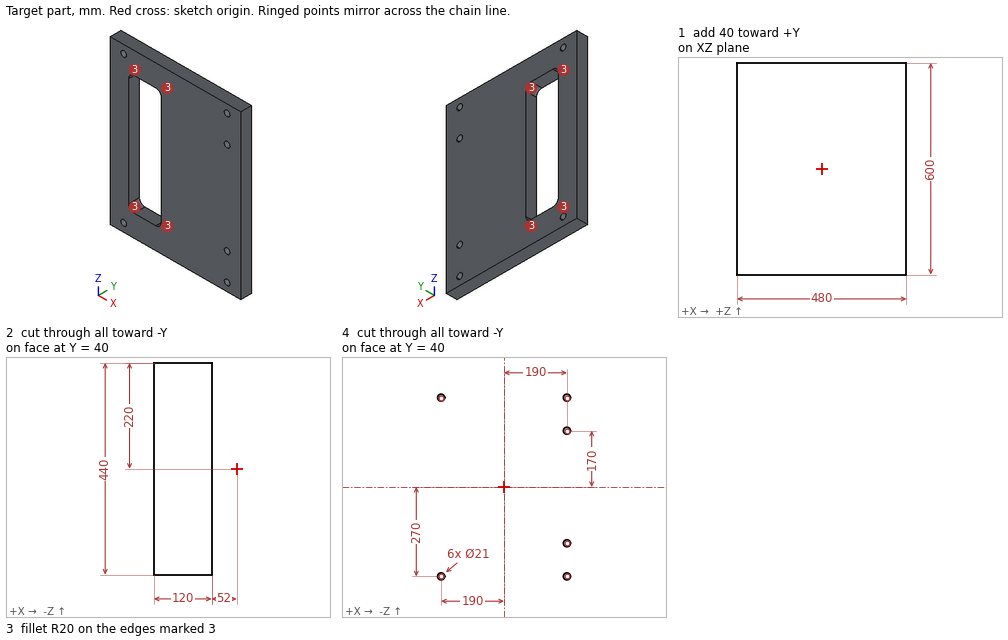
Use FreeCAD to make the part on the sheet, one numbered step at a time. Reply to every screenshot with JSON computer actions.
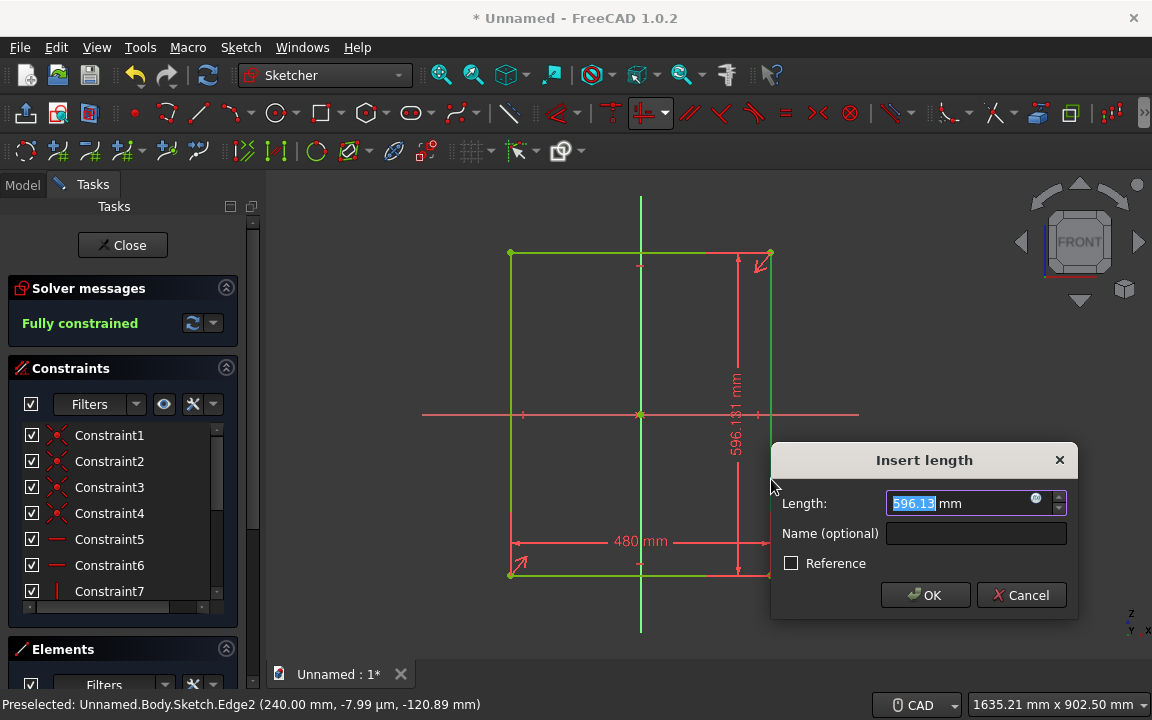
{"action": "type", "text": "600"}
{"action": "key", "text": "Return"}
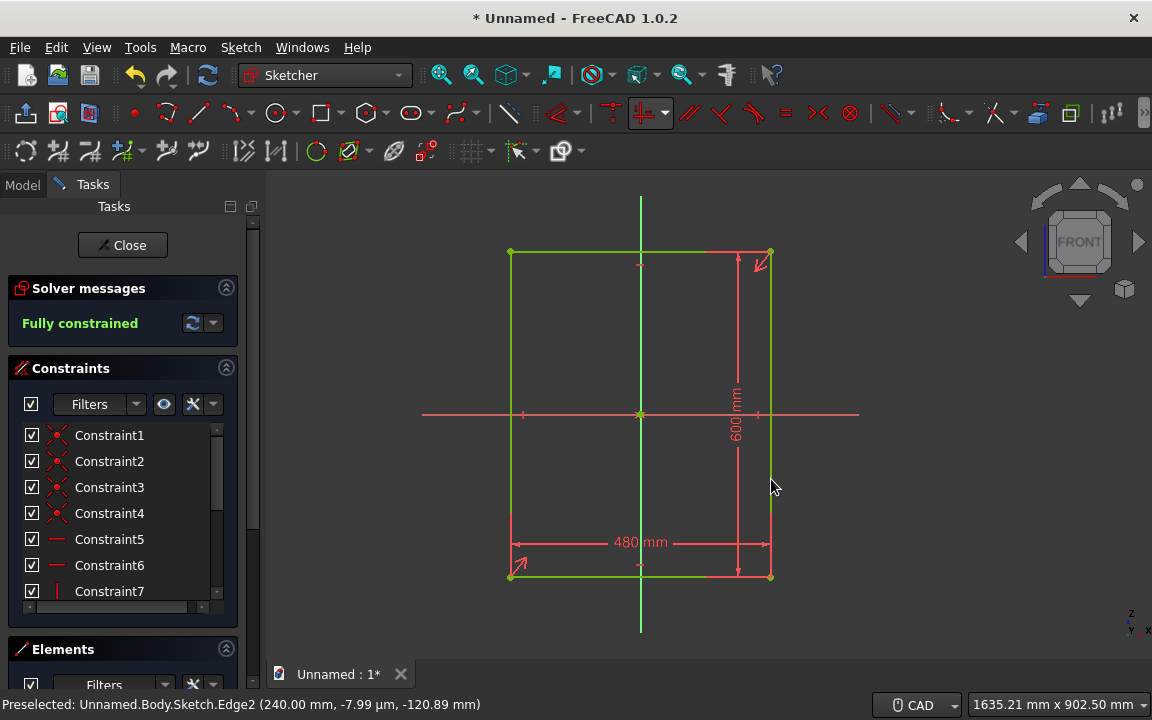
{"action": "left_click", "coordinate": [123, 245]}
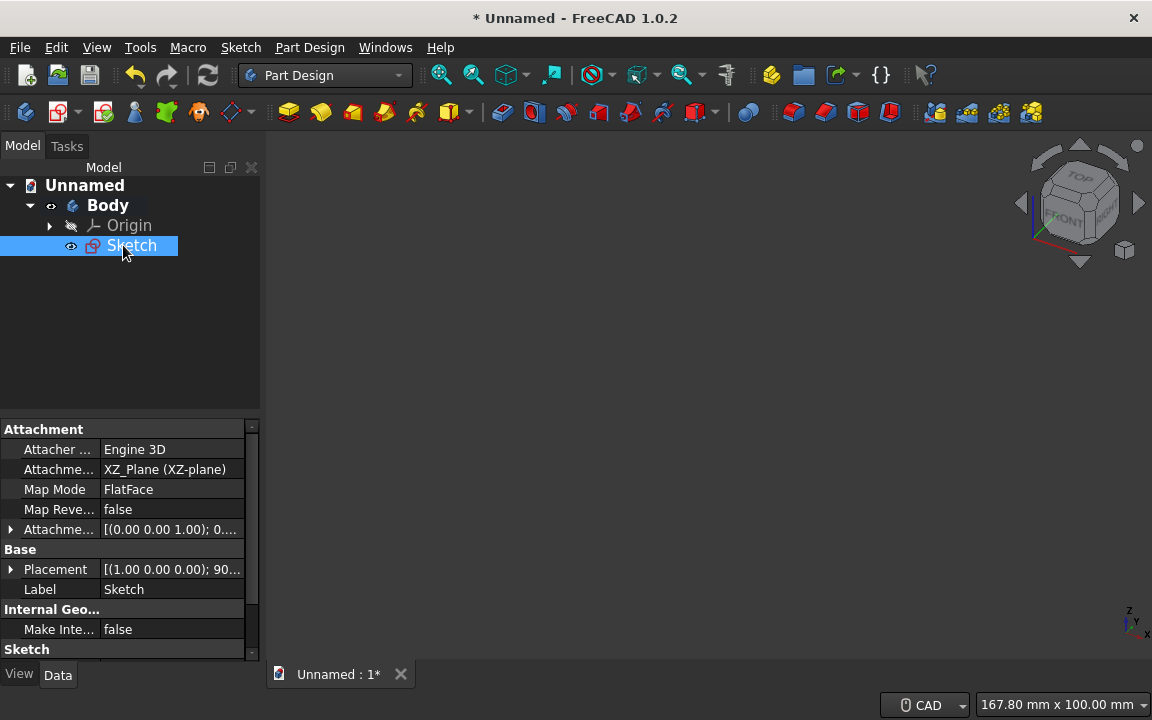
{"action": "left_click", "coordinate": [290, 112]}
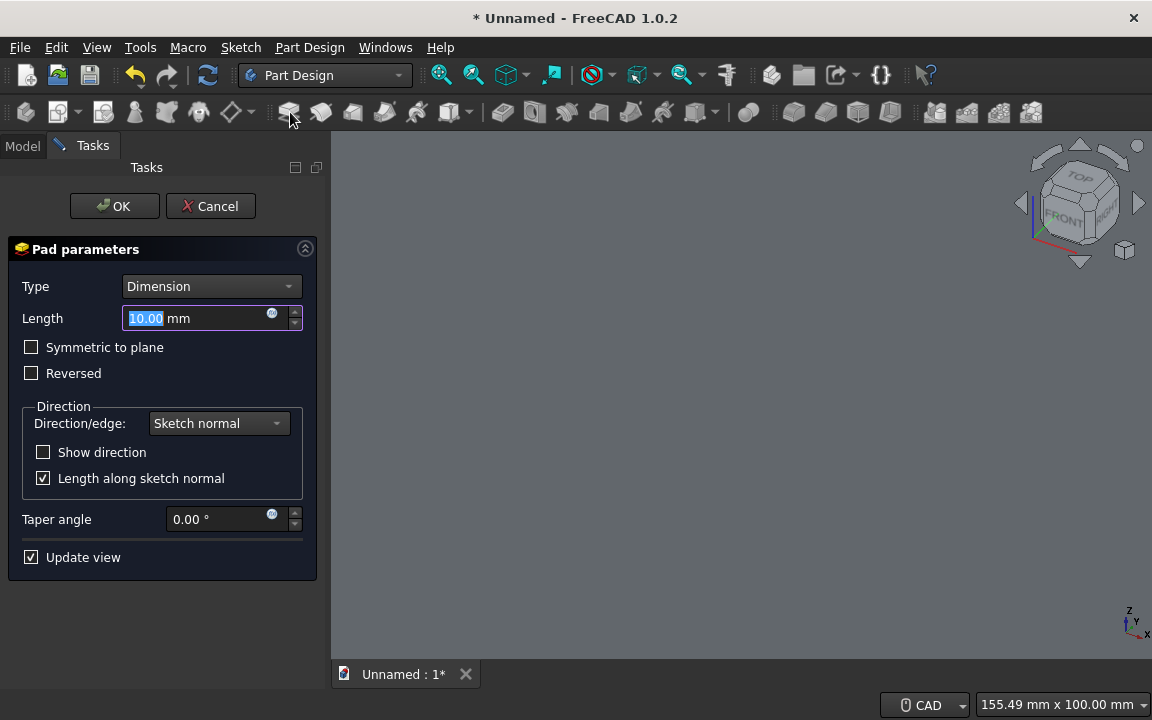
{"action": "type", "text": "40"}
{"action": "key", "text": "Tab"}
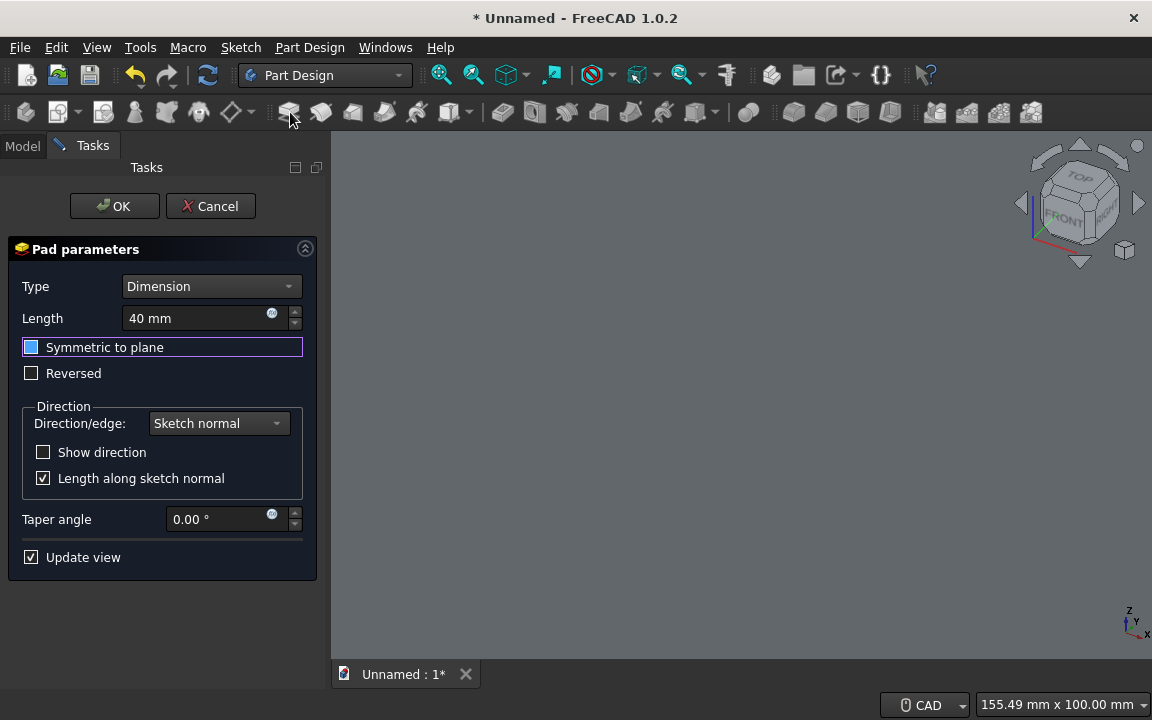
{"action": "left_click", "coordinate": [30, 373]}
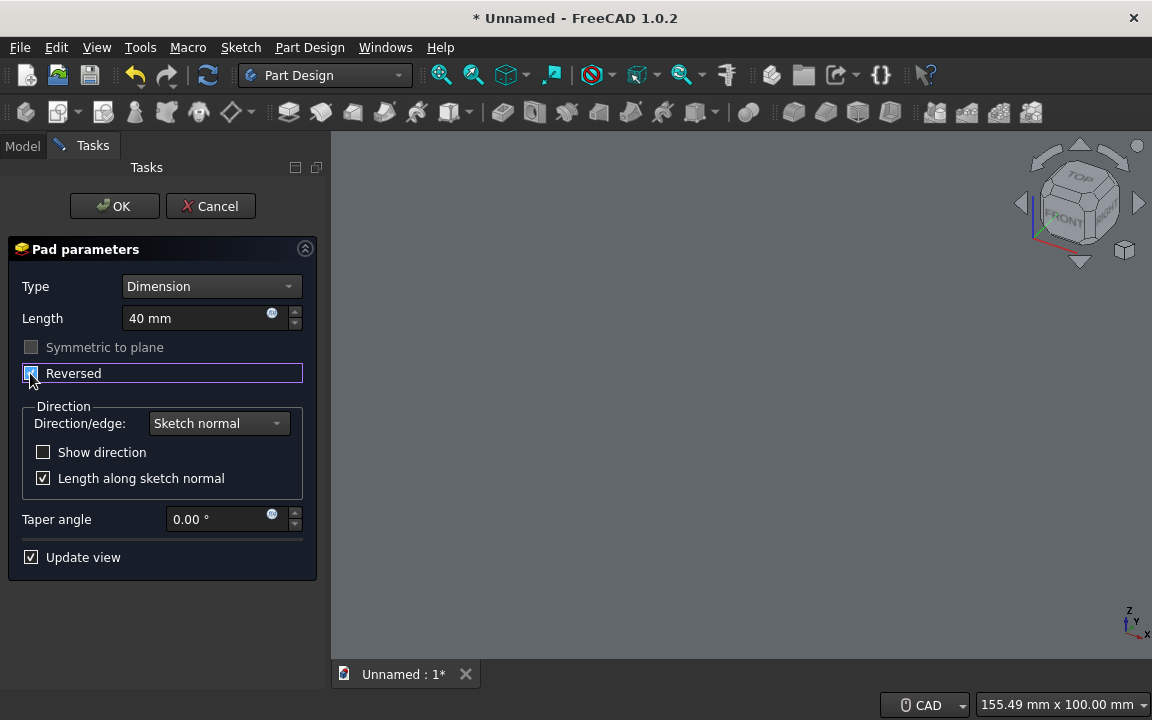
{"action": "left_click", "coordinate": [115, 206]}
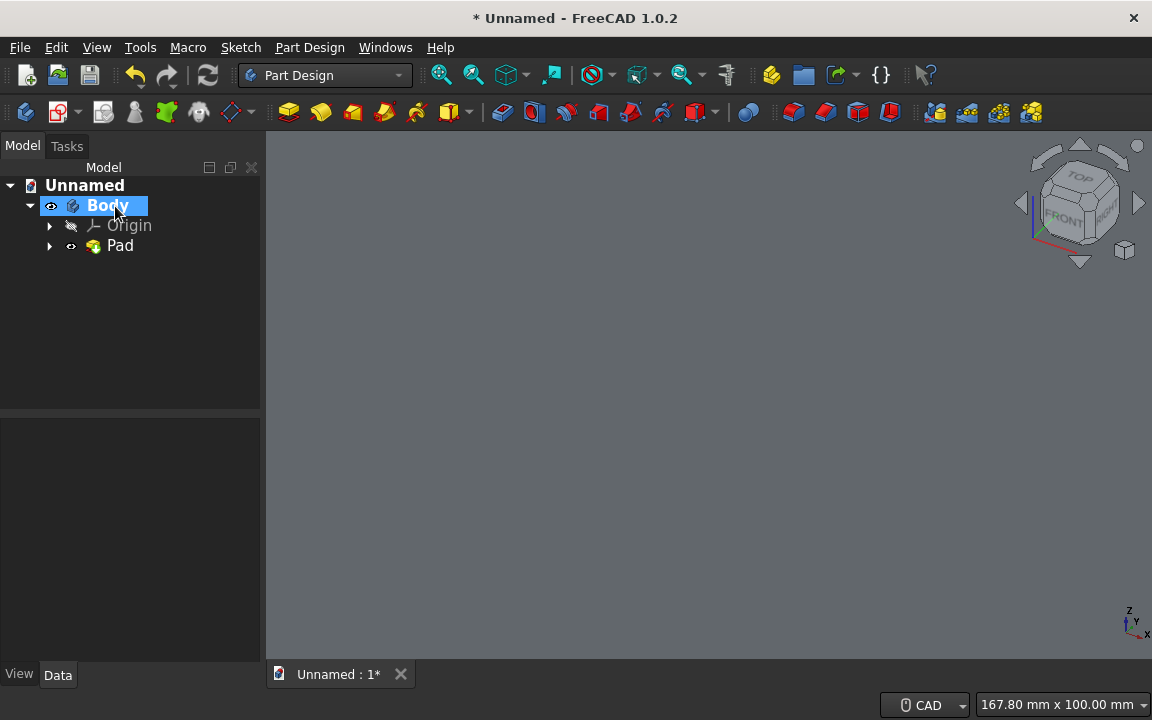
{"action": "key", "text": "v f"}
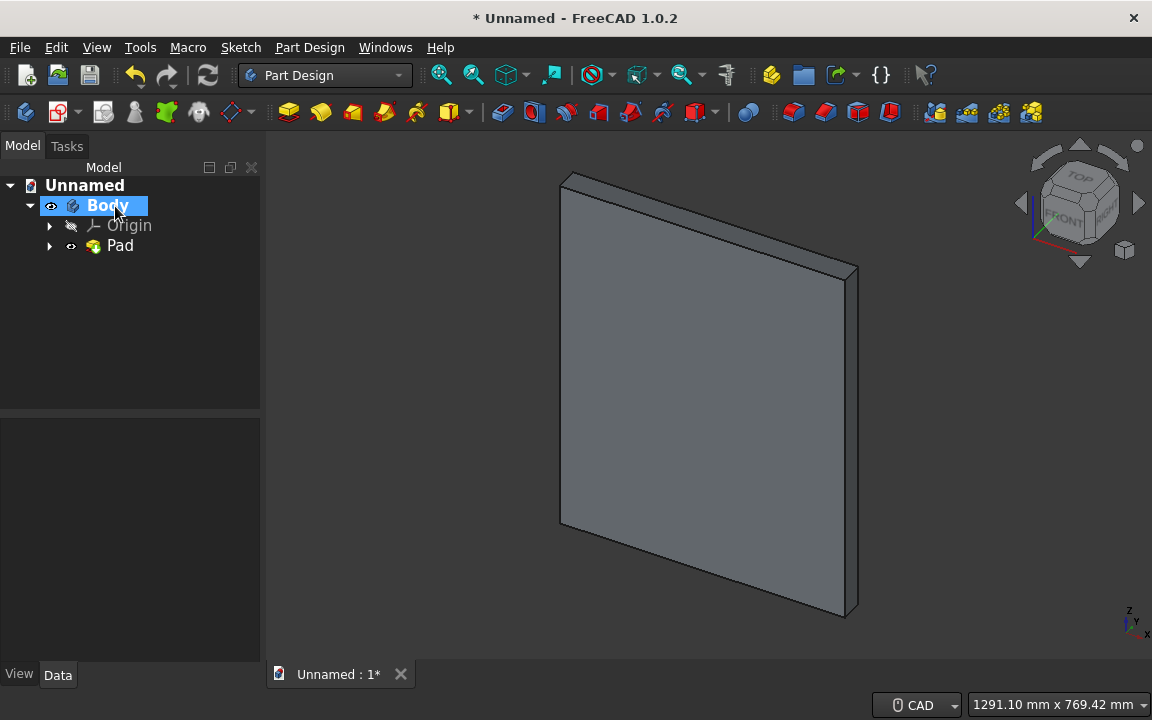
{"action": "key", "text": "4"}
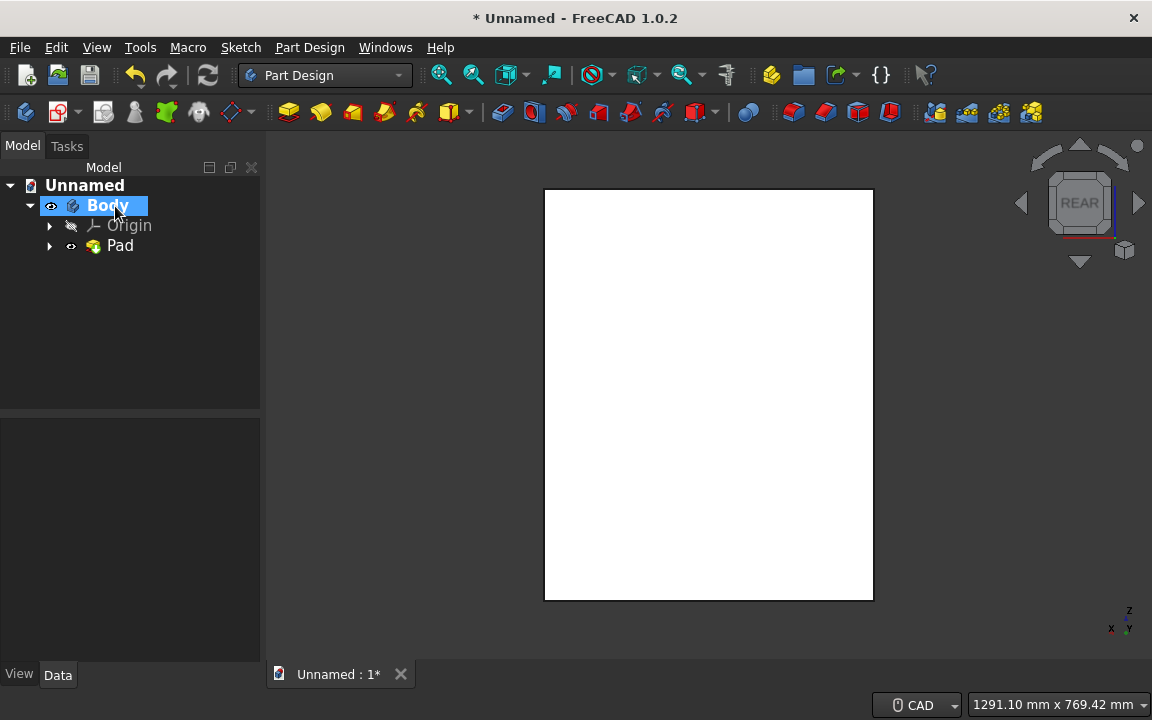
{"action": "left_click", "coordinate": [709, 394]}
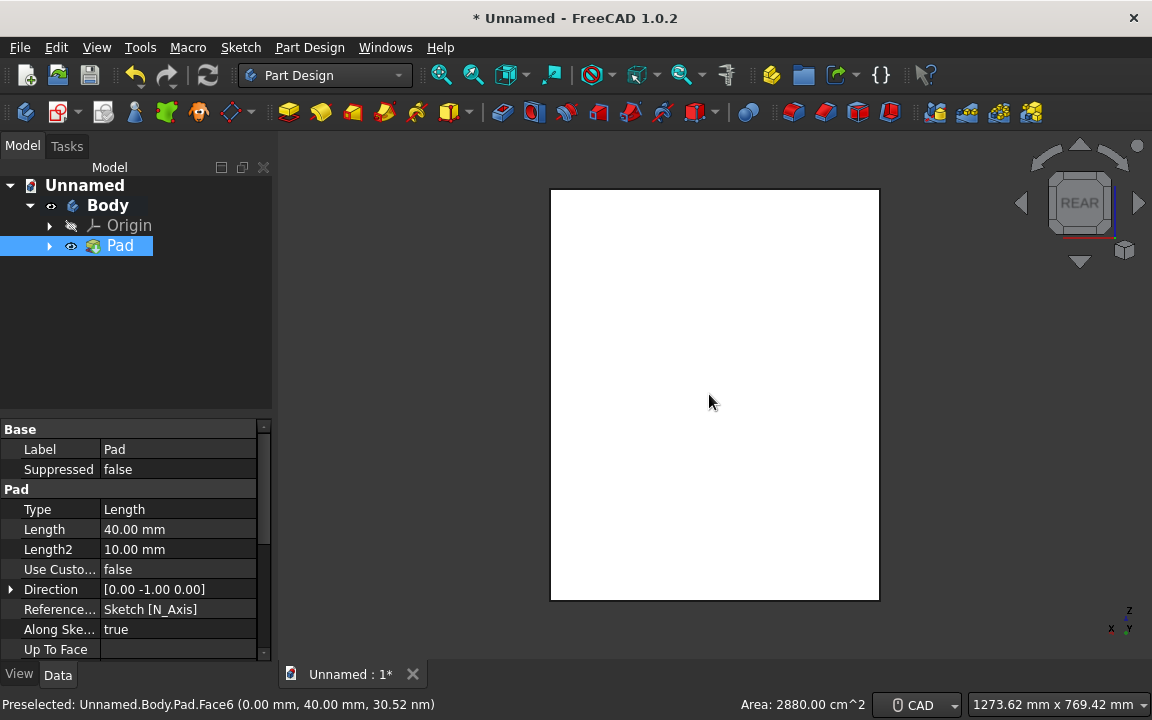
{"action": "left_click", "coordinate": [58, 112]}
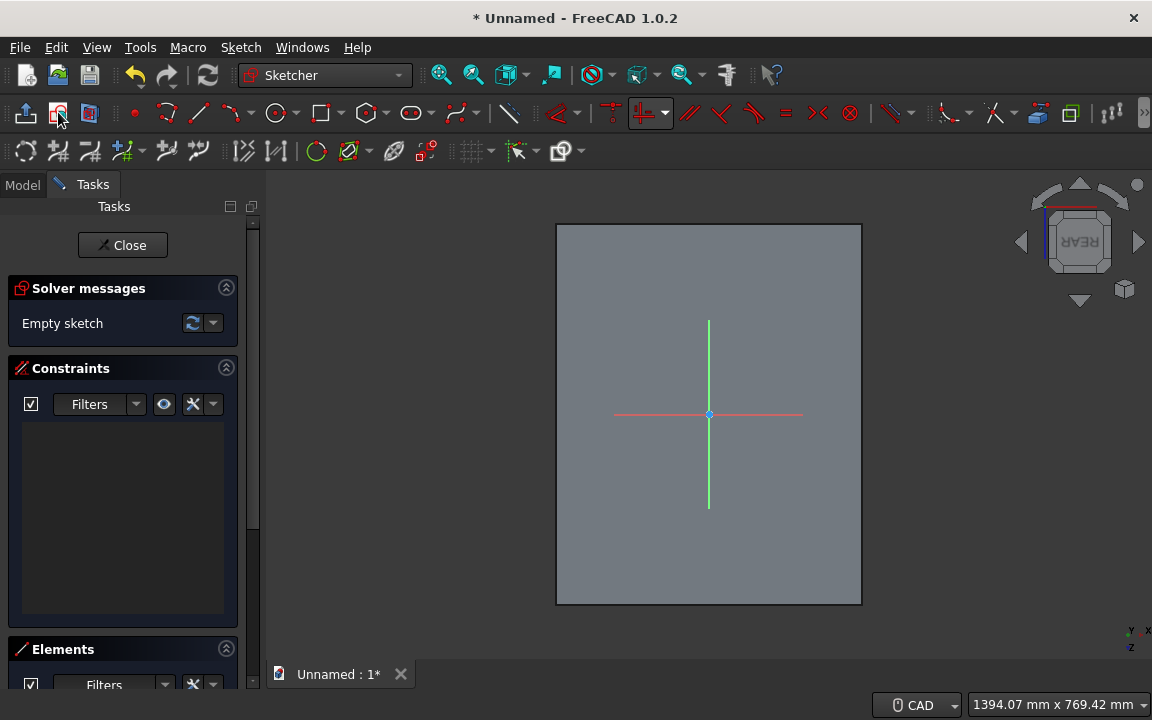
{"action": "left_click", "coordinate": [322, 114]}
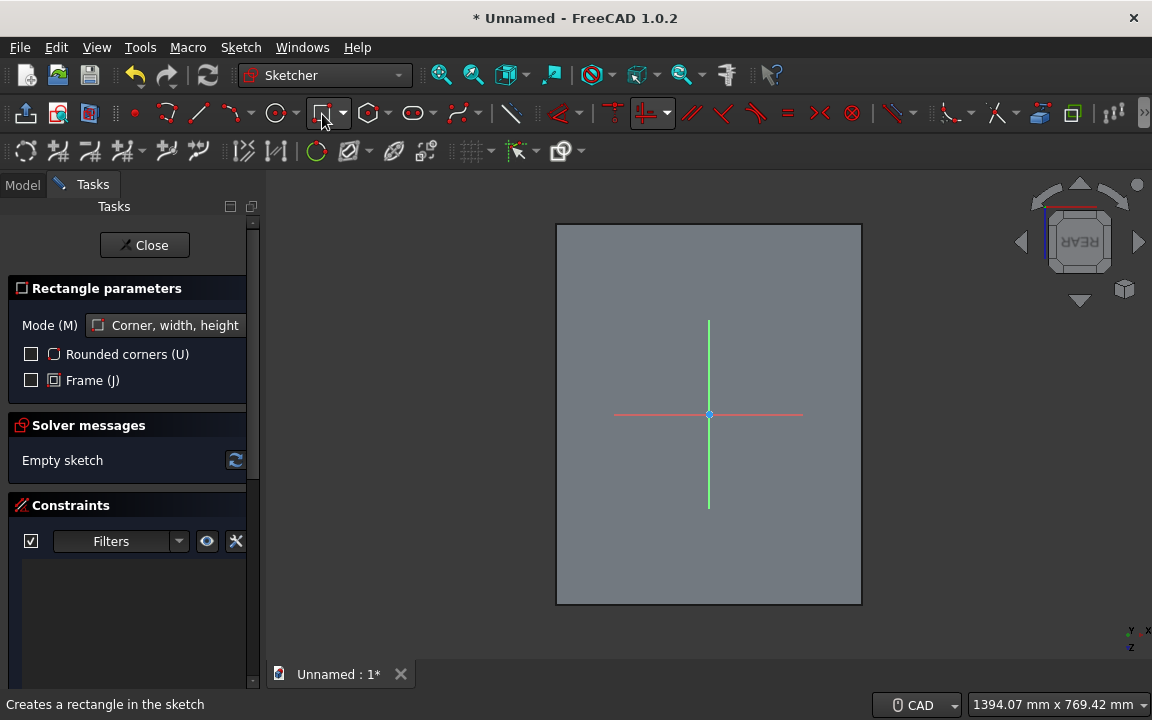
{"action": "left_click", "coordinate": [600, 275]}
{"action": "left_click", "coordinate": [676, 554]}
{"action": "key", "text": "Escape"}